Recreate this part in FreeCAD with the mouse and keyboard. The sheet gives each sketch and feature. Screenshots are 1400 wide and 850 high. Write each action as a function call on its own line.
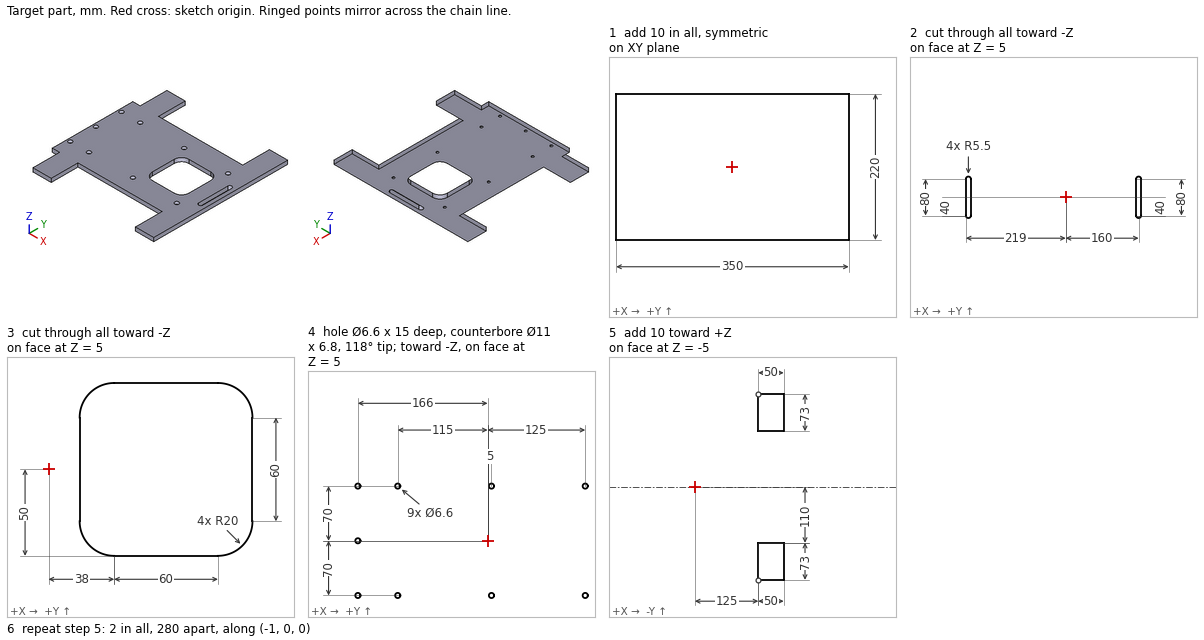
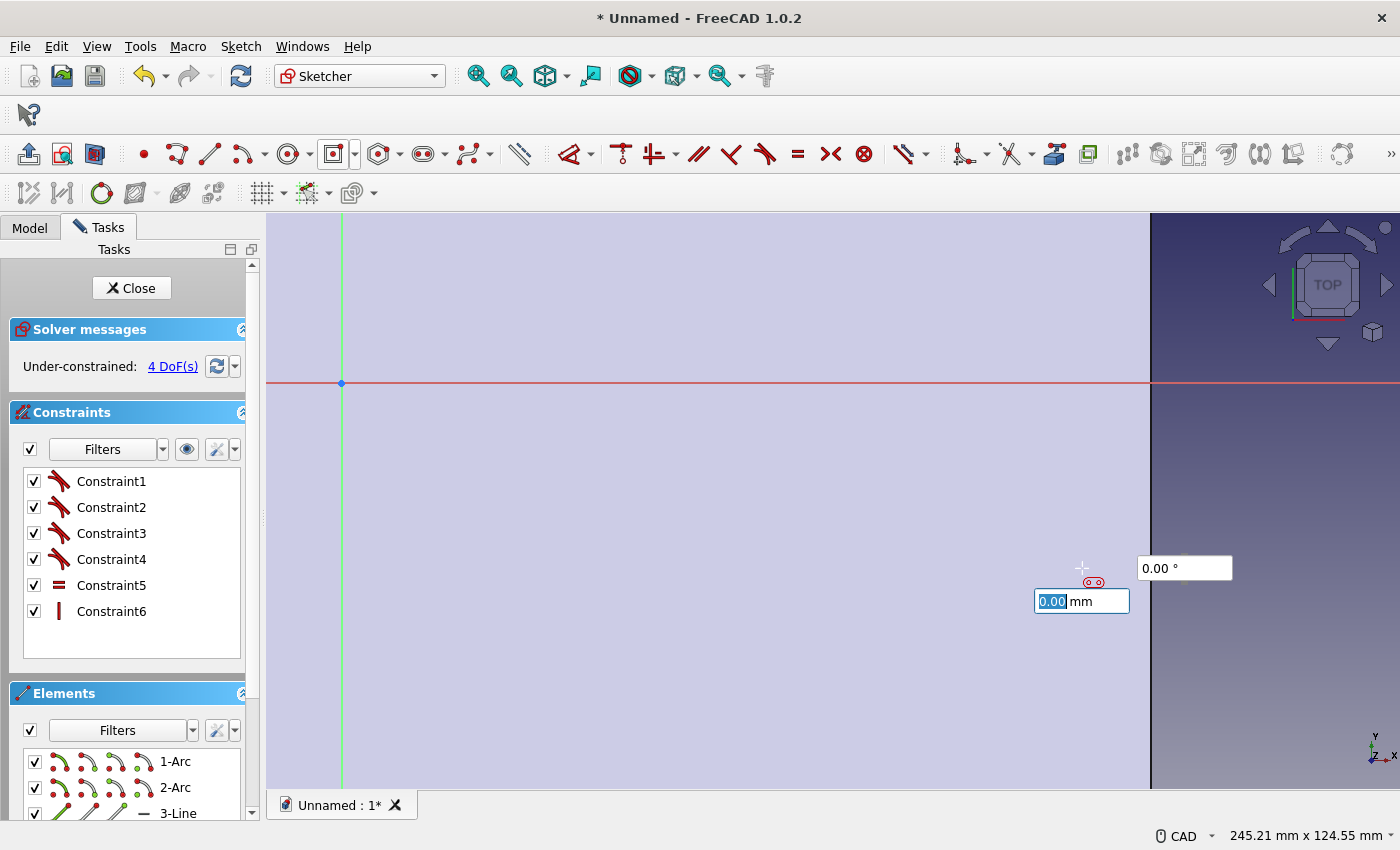
scroll(1083, 569, down, 5)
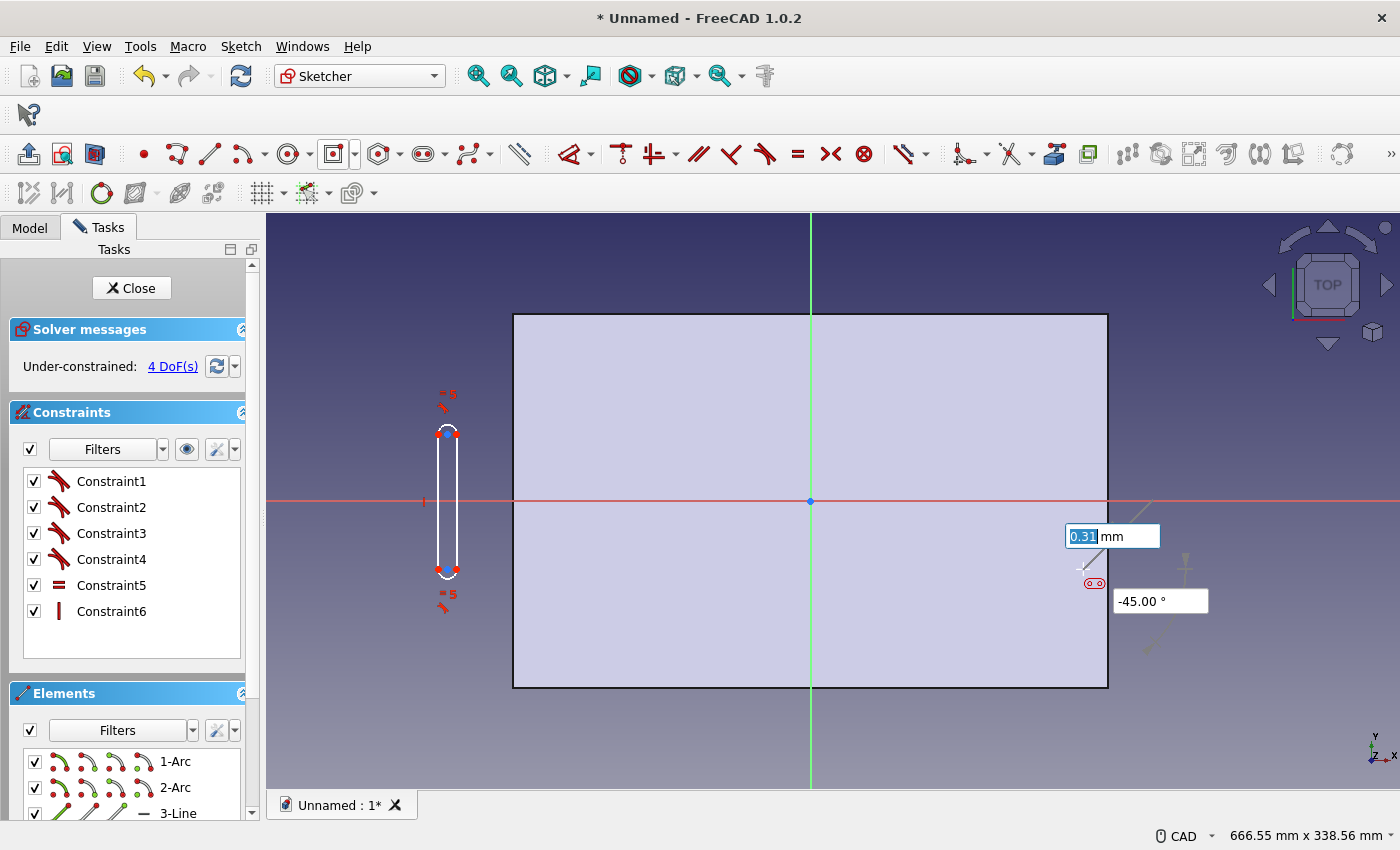
click(1083, 433)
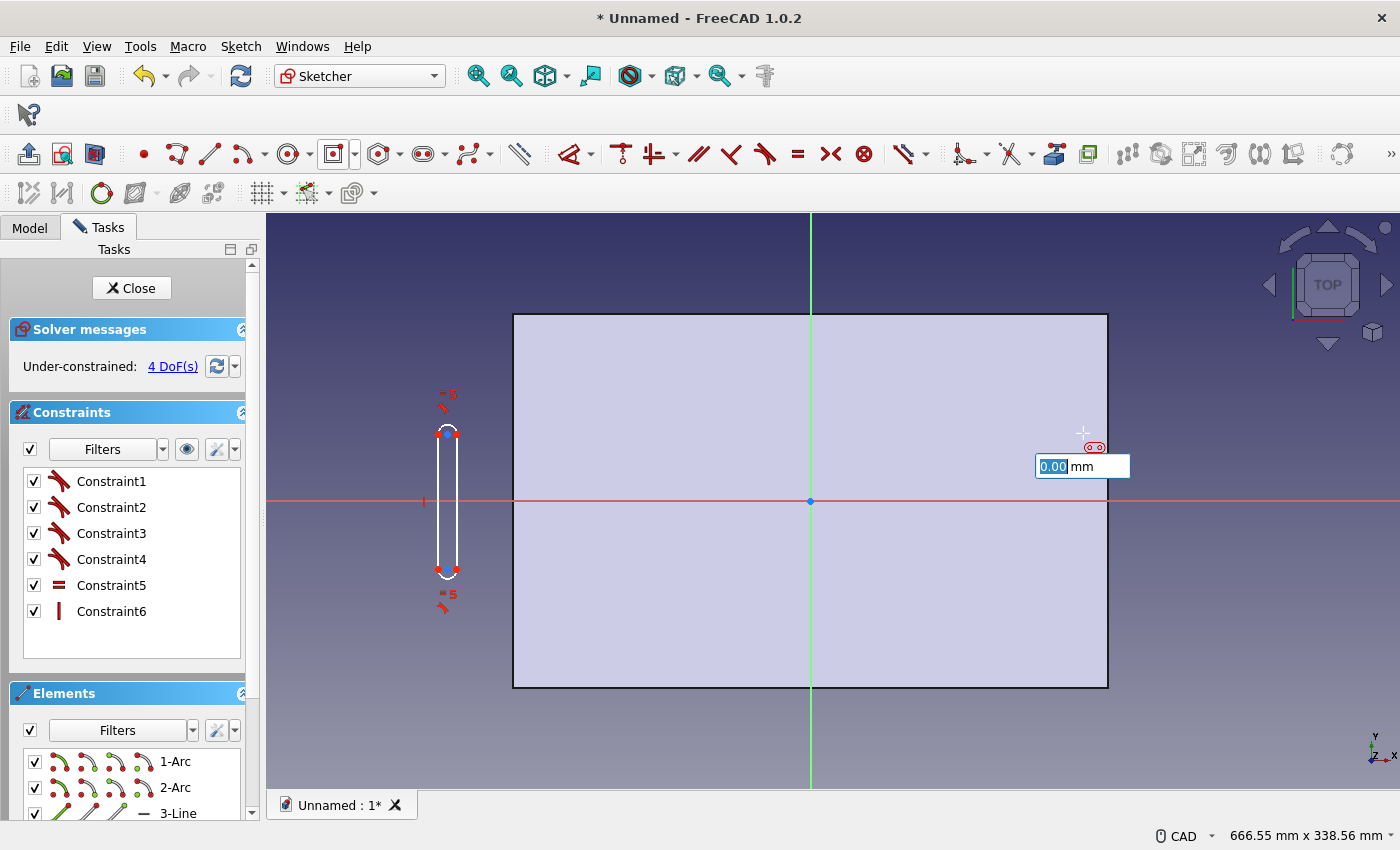
scroll(1092, 522, up, 3)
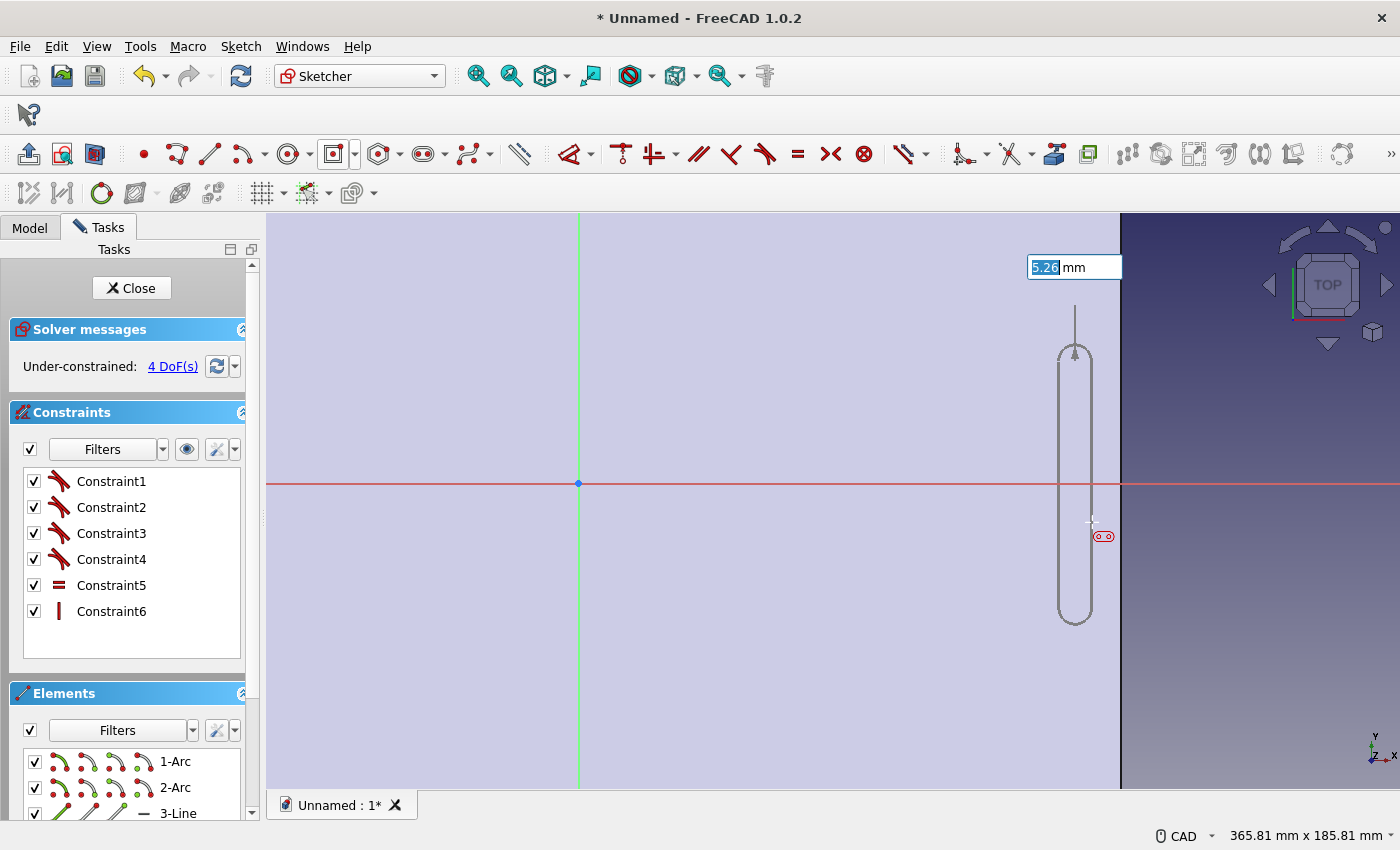
click(1092, 521)
key(Escape)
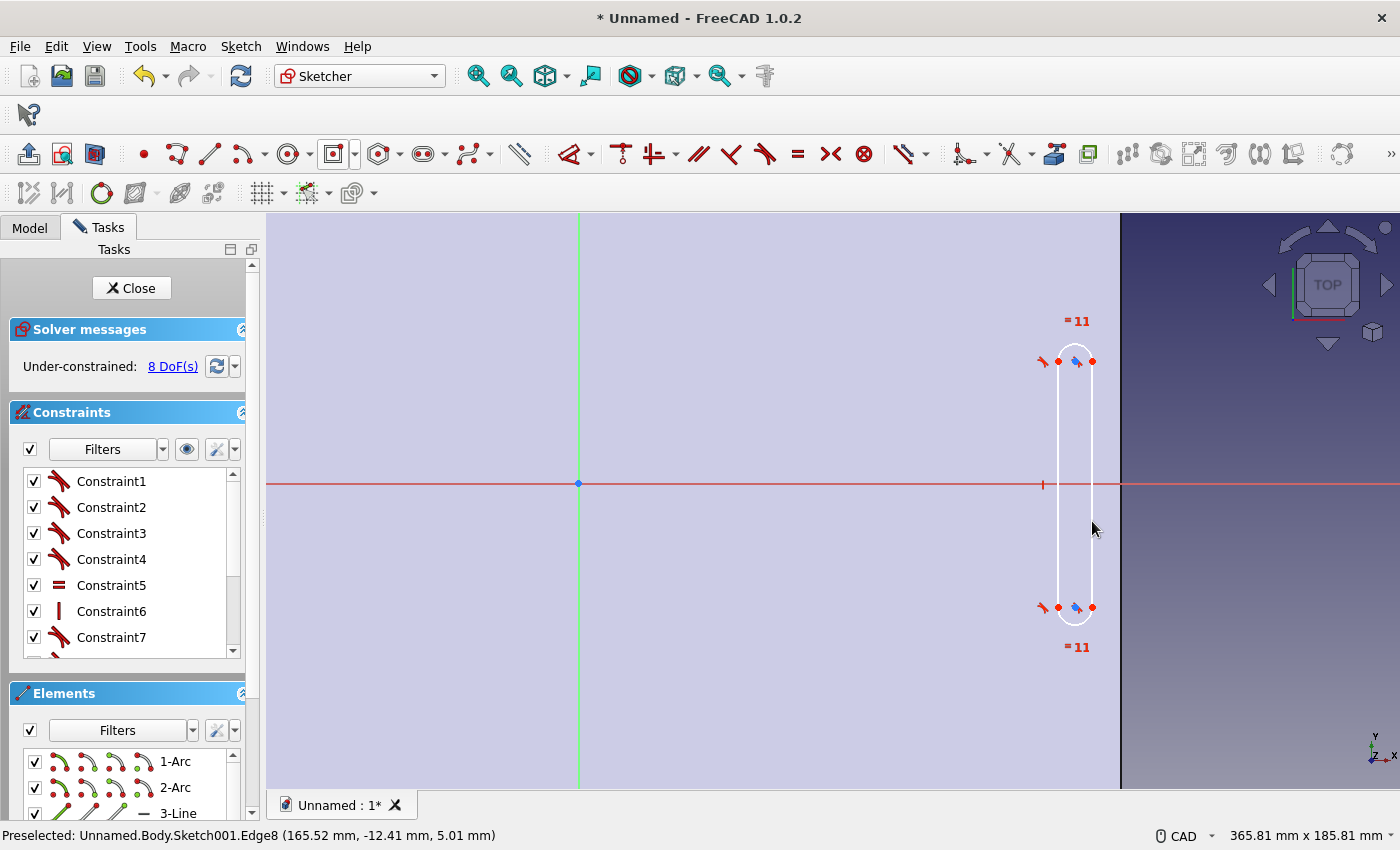
scroll(1091, 522, down, 3)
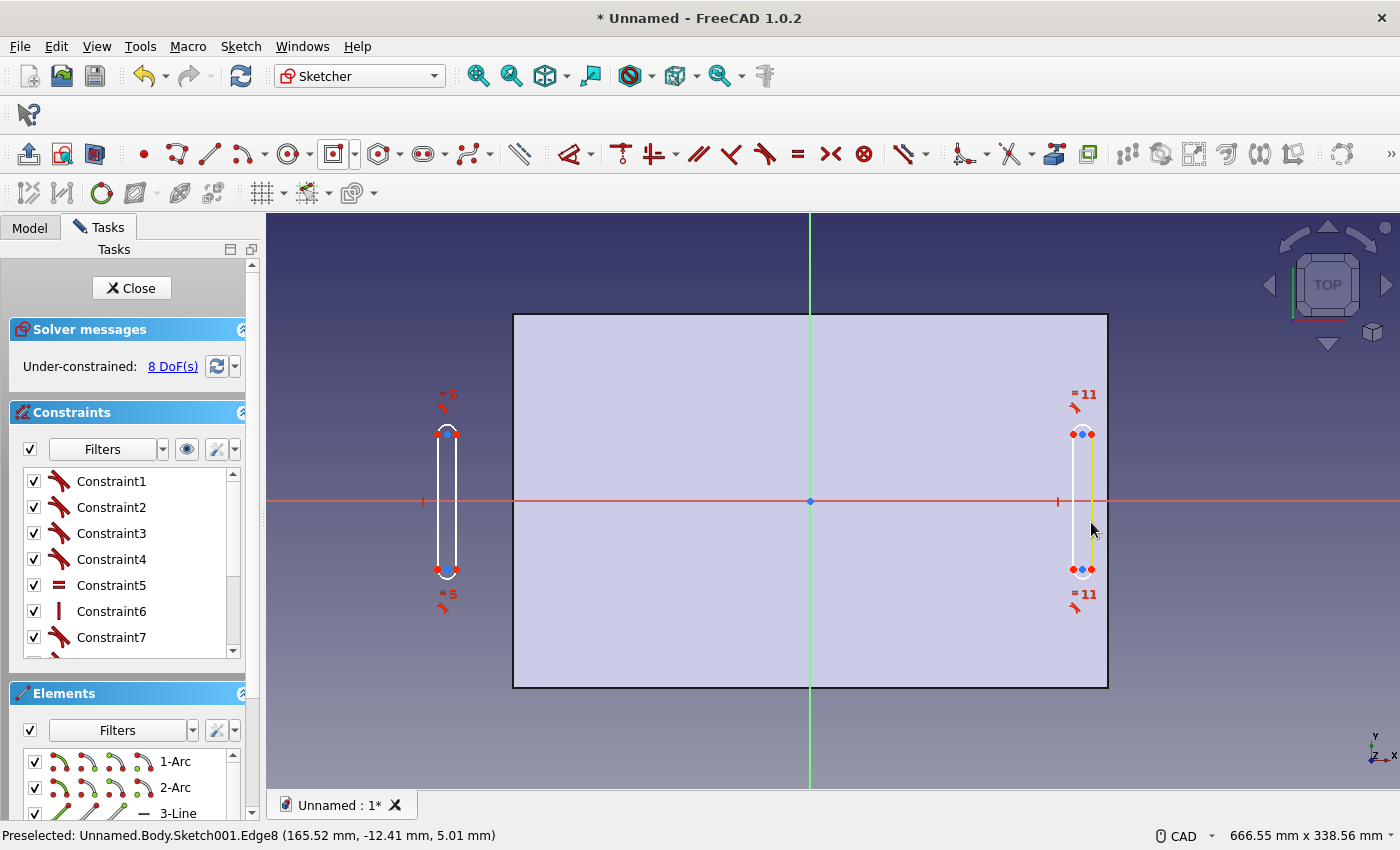
scroll(442, 577, up, 3)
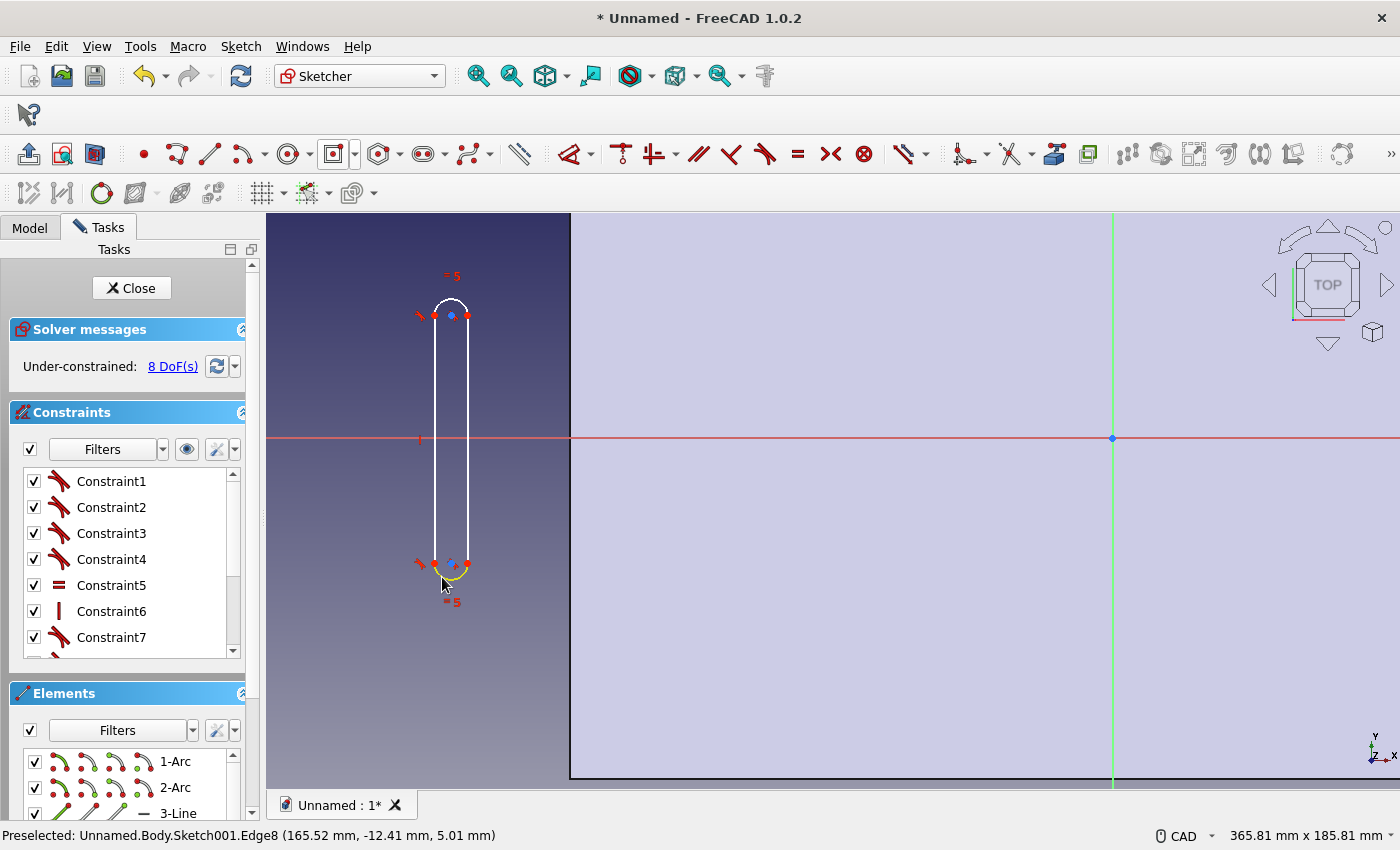
click(441, 577)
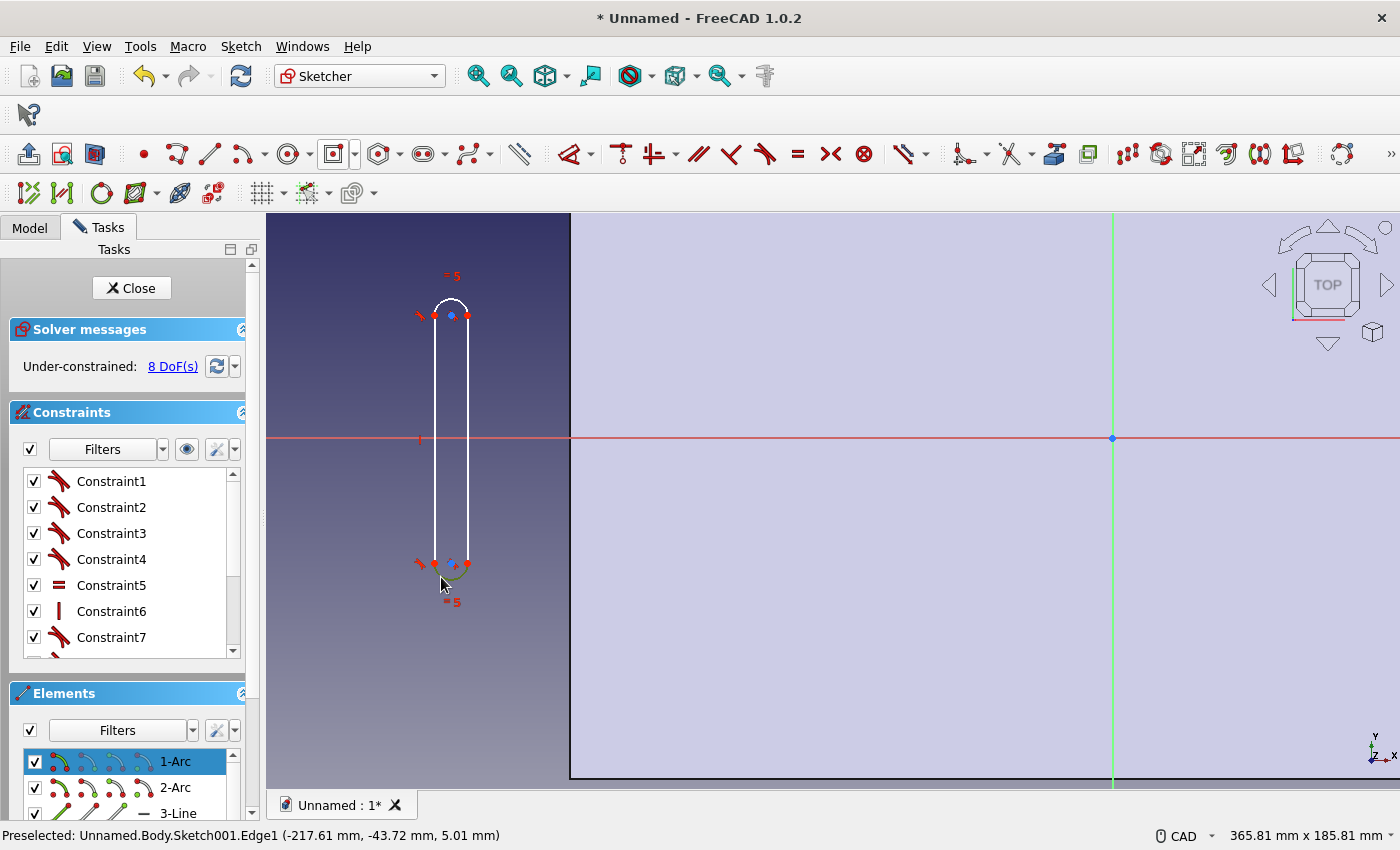
scroll(441, 577, down, 3)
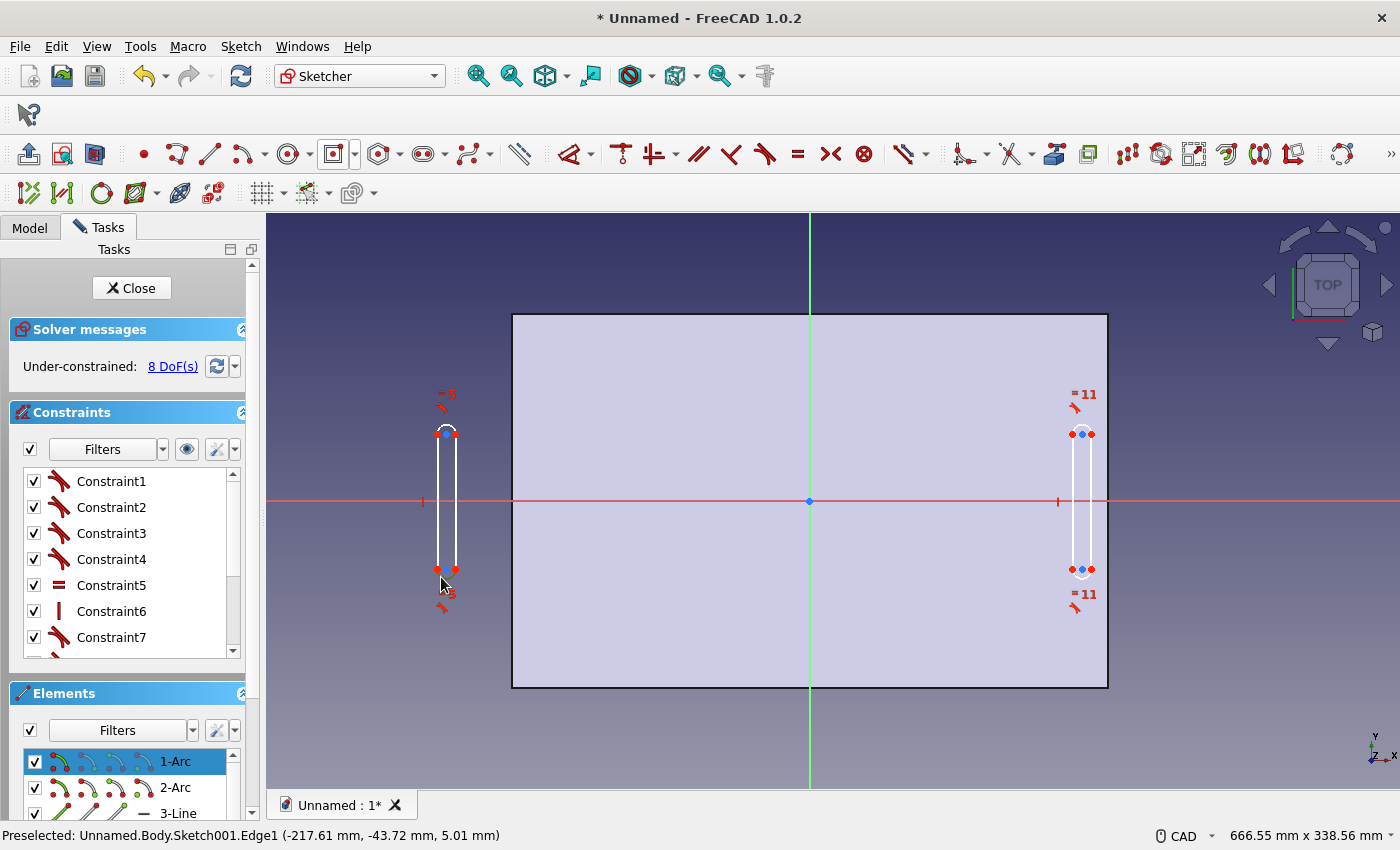
scroll(1077, 577, up, 3)